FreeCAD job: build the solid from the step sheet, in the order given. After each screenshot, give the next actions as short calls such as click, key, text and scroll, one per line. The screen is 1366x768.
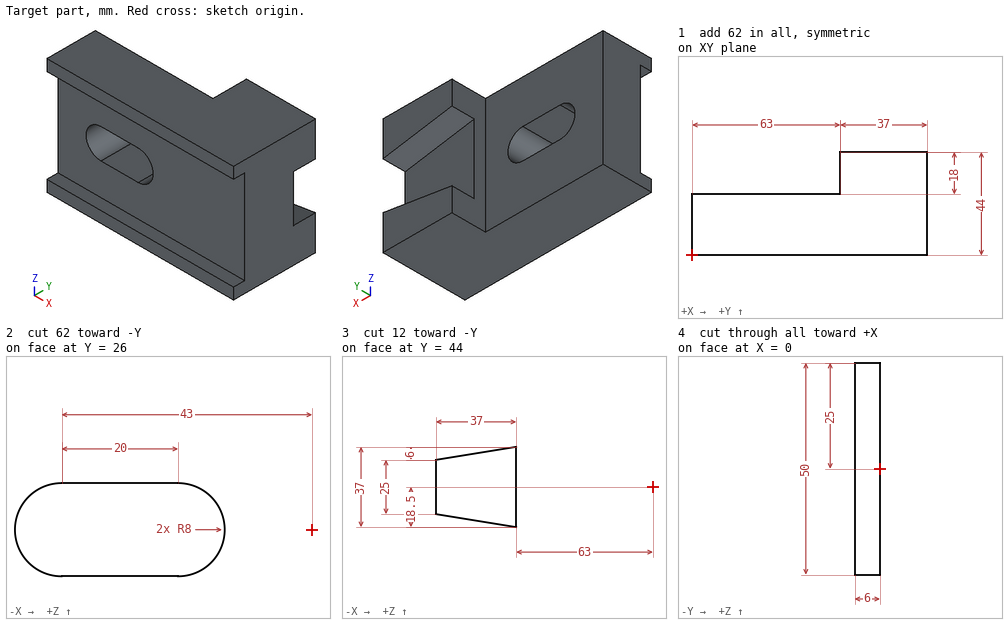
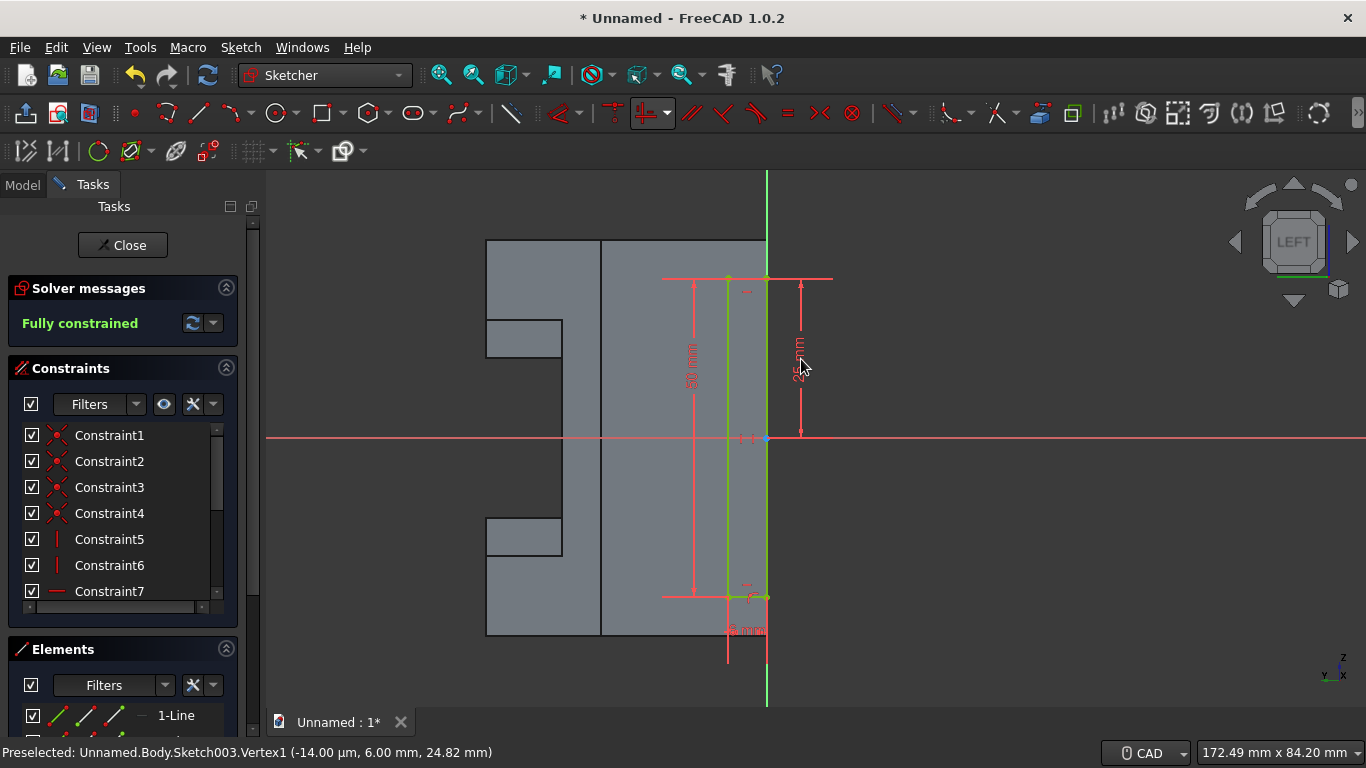
click(123, 245)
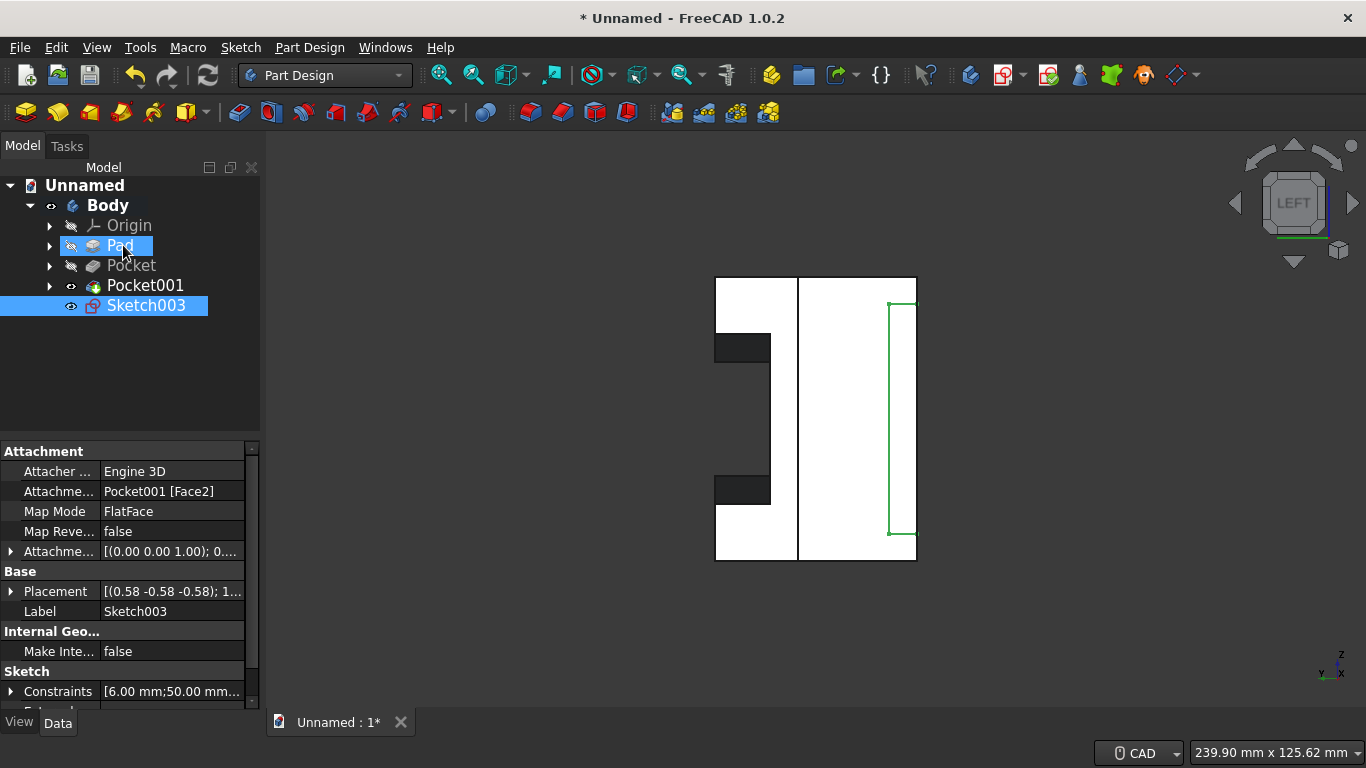
click(240, 112)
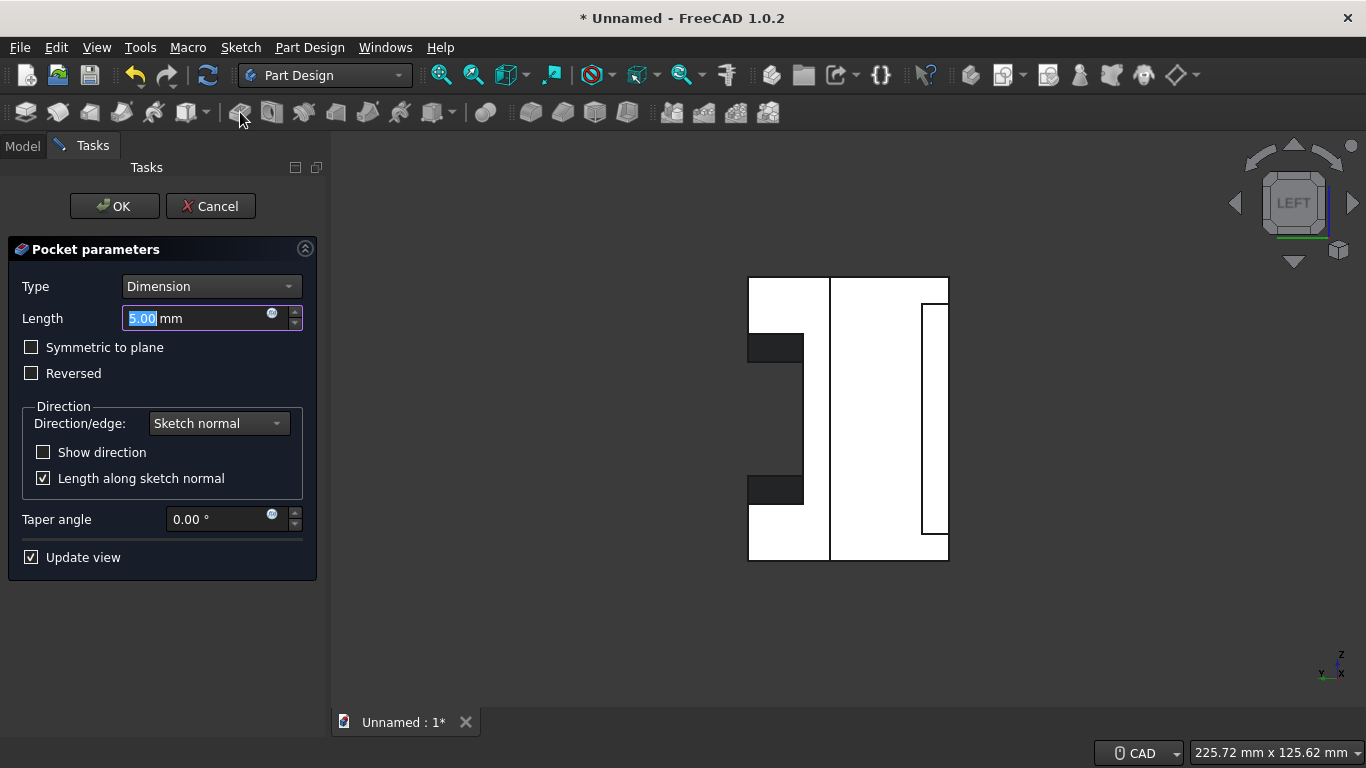
click(212, 286)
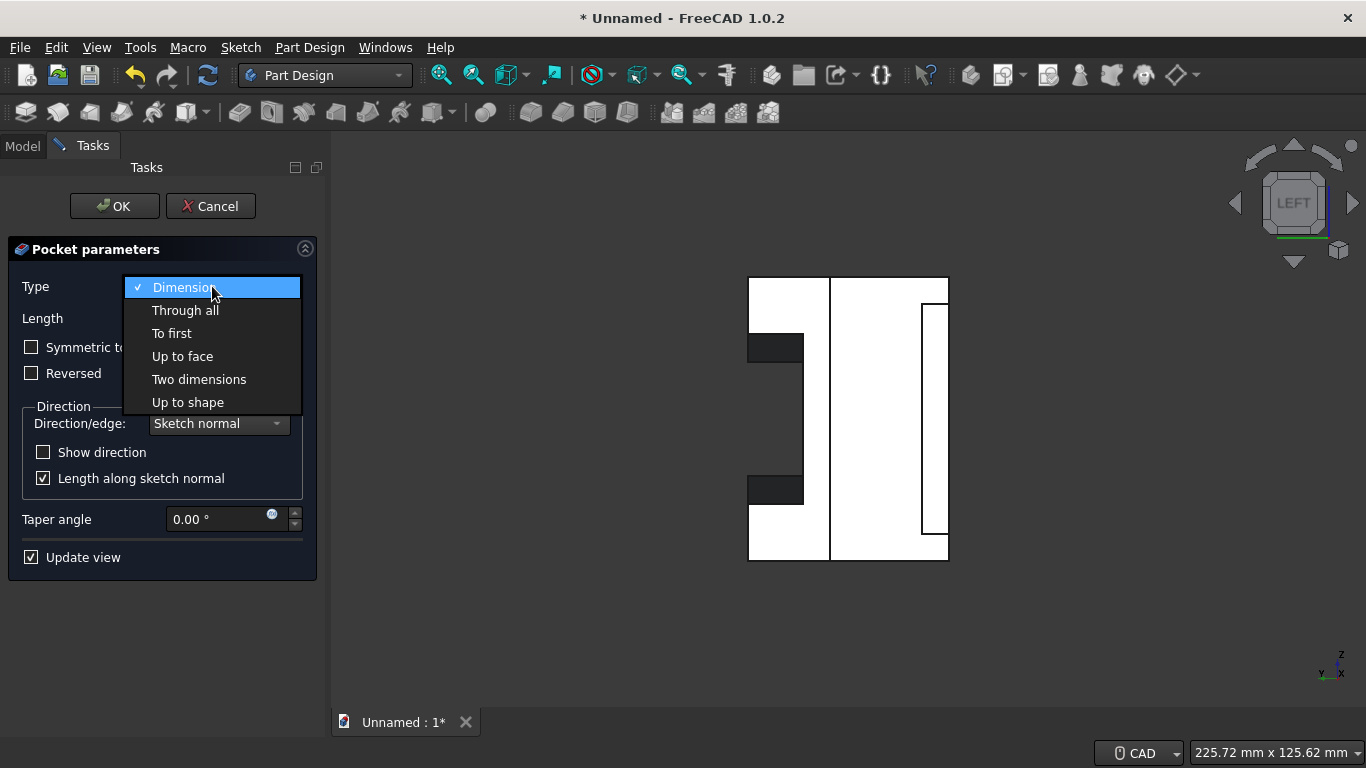
click(212, 310)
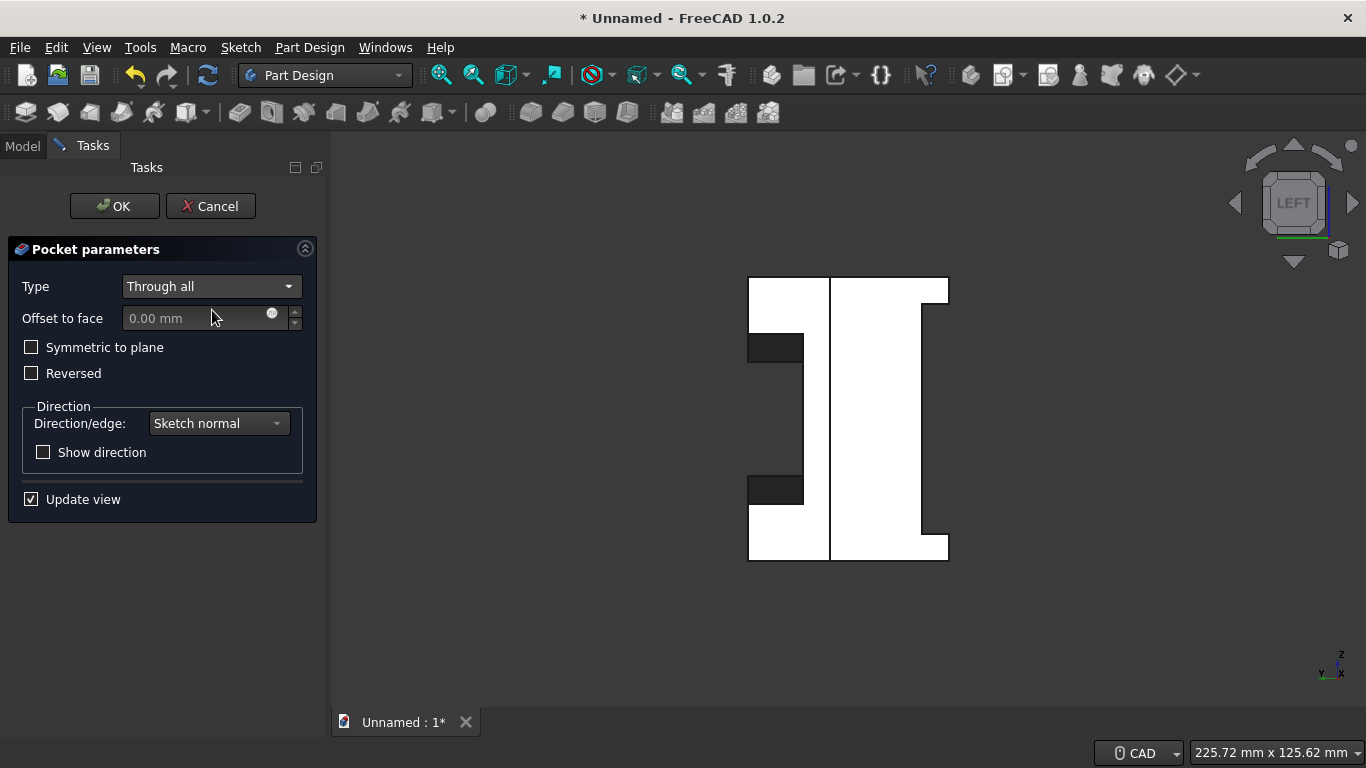
click(115, 206)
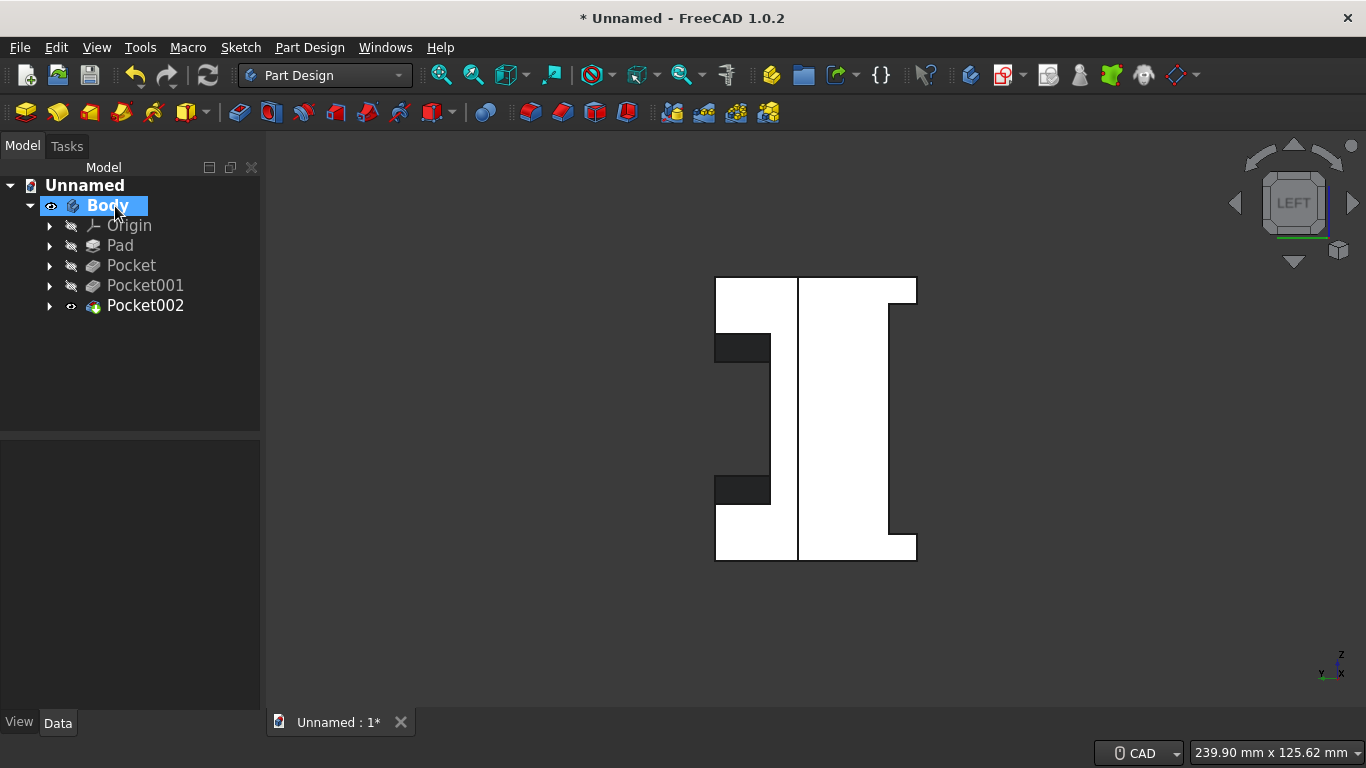
key(0)